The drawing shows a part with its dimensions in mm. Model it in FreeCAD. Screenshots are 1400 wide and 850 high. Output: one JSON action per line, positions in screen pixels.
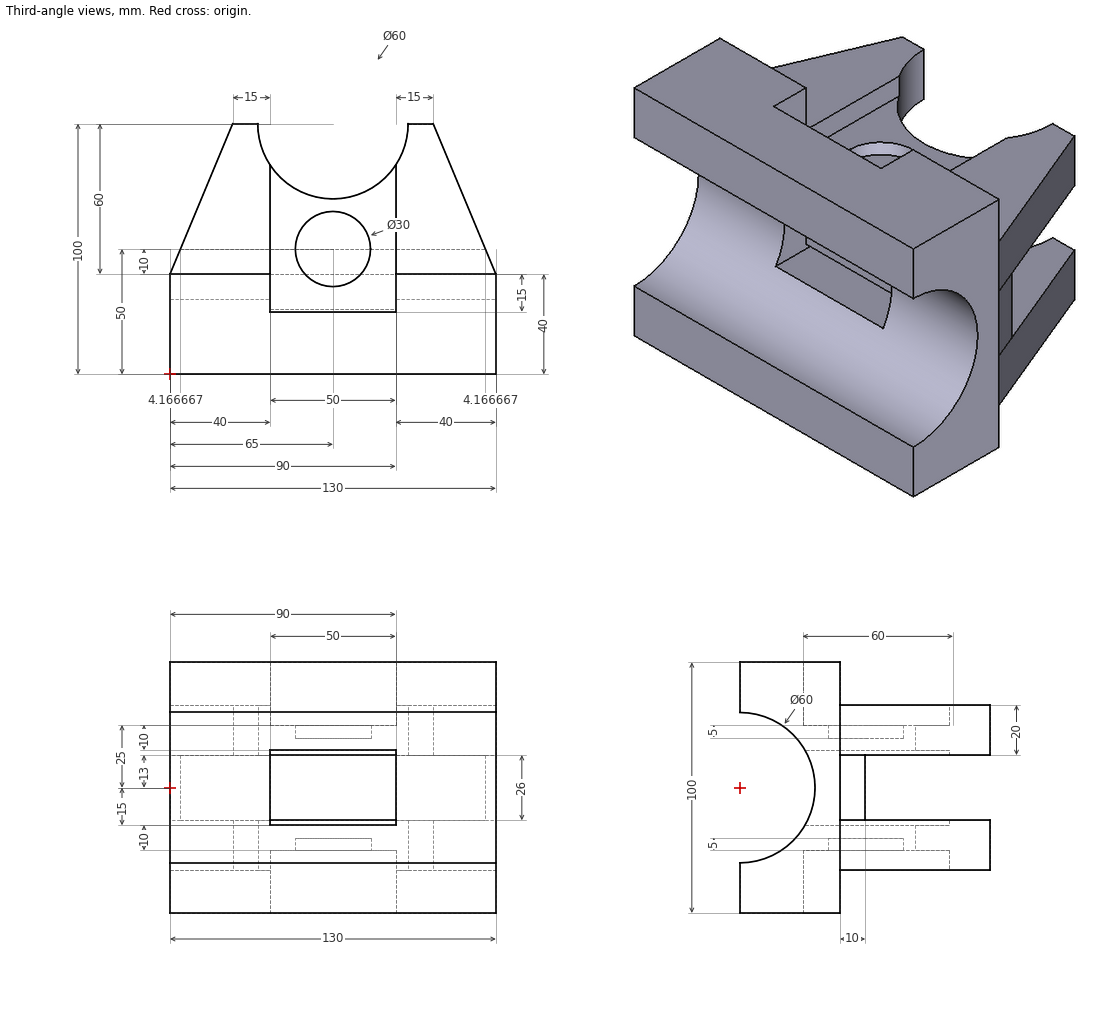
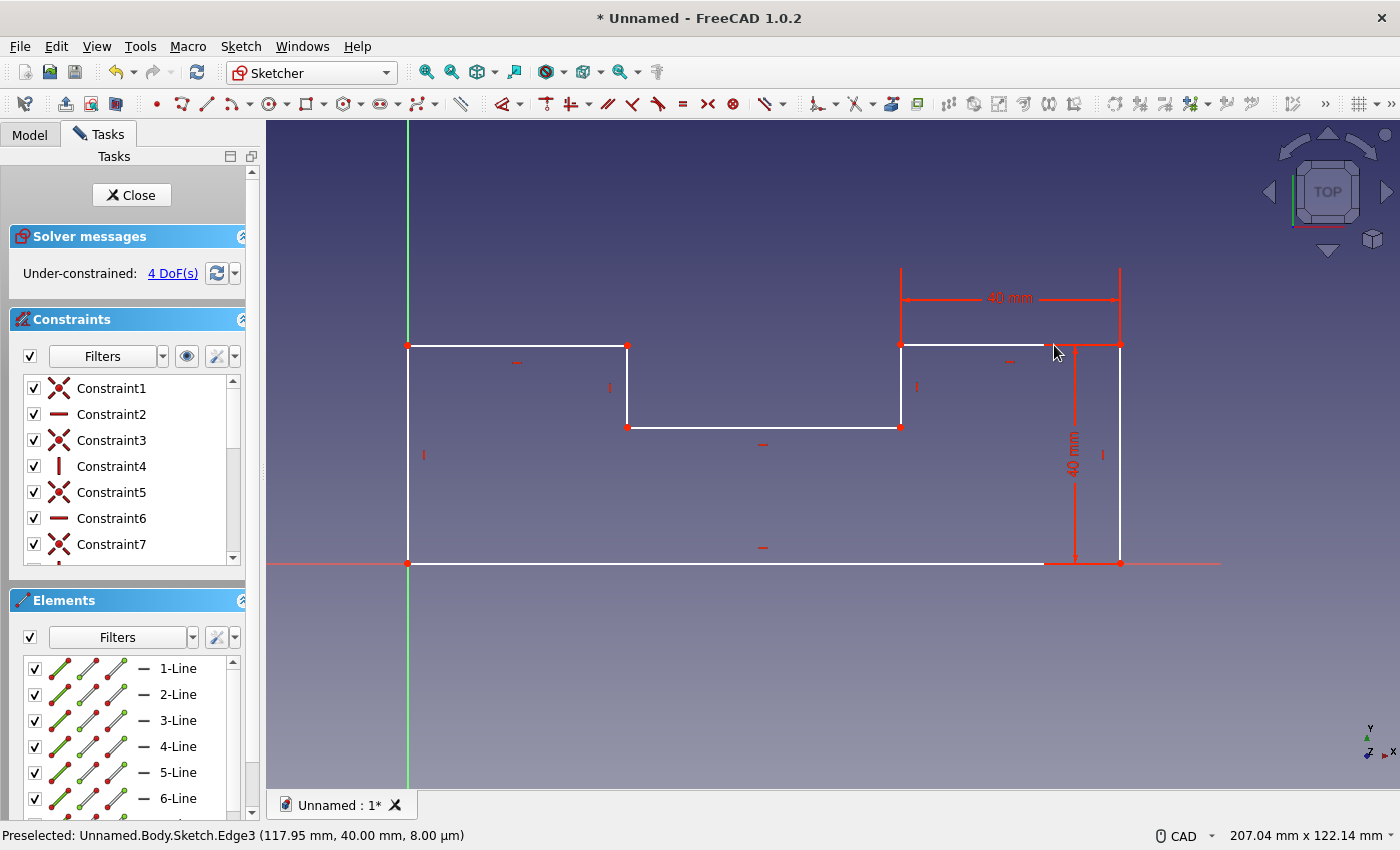
{"action": "left_click", "coordinate": [901, 370]}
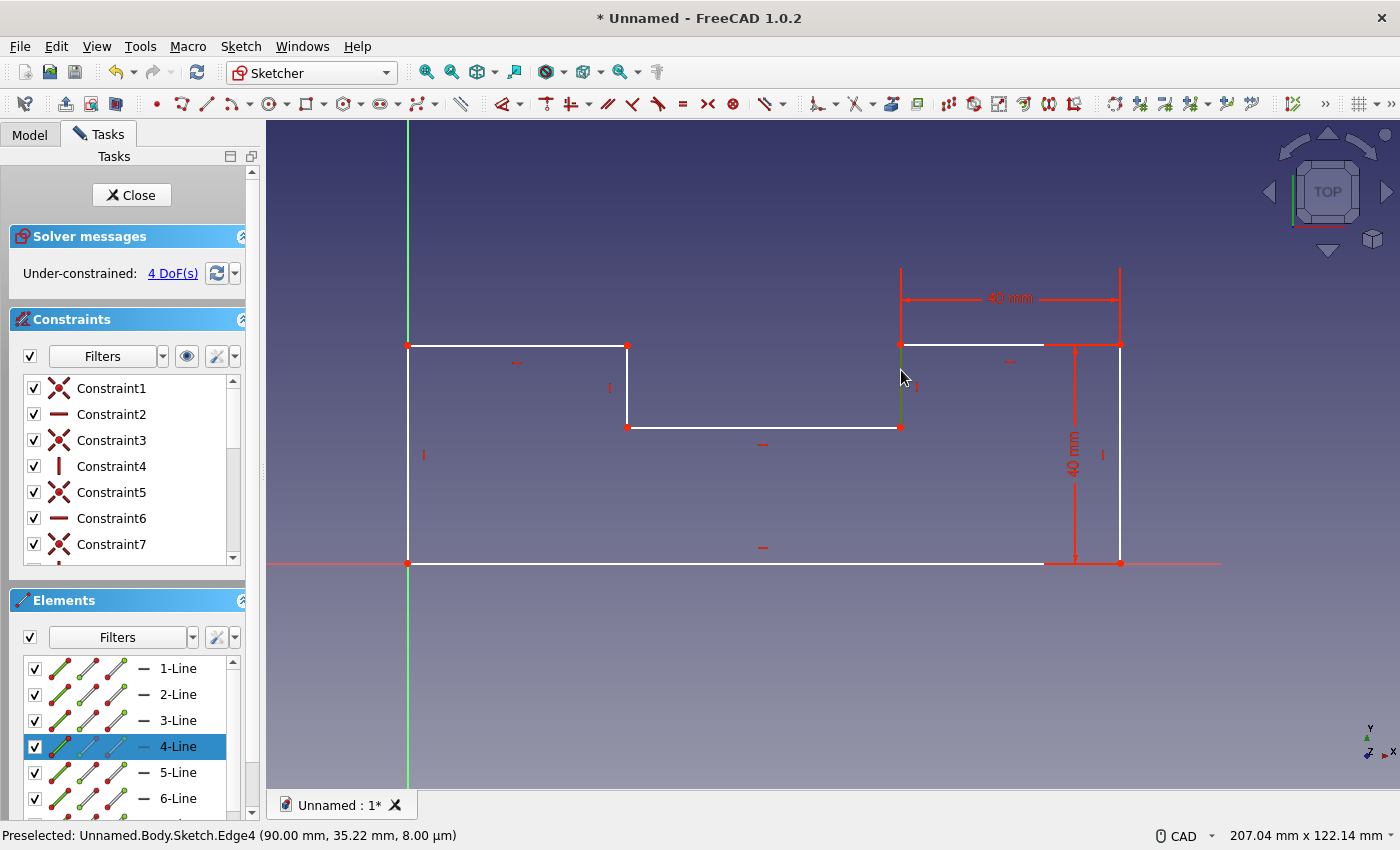
{"action": "left_click", "coordinate": [520, 104]}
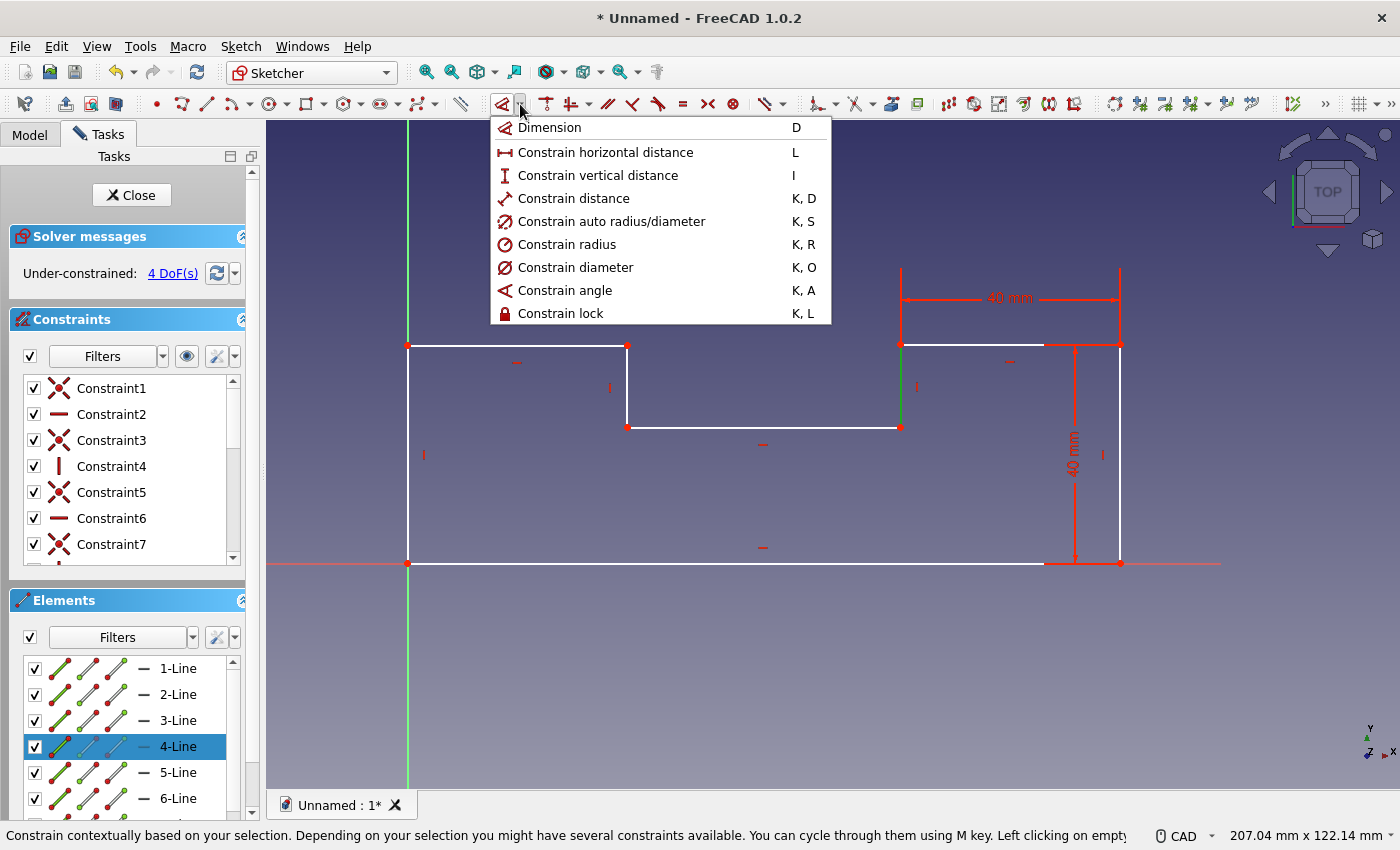
{"action": "left_click", "coordinate": [661, 176]}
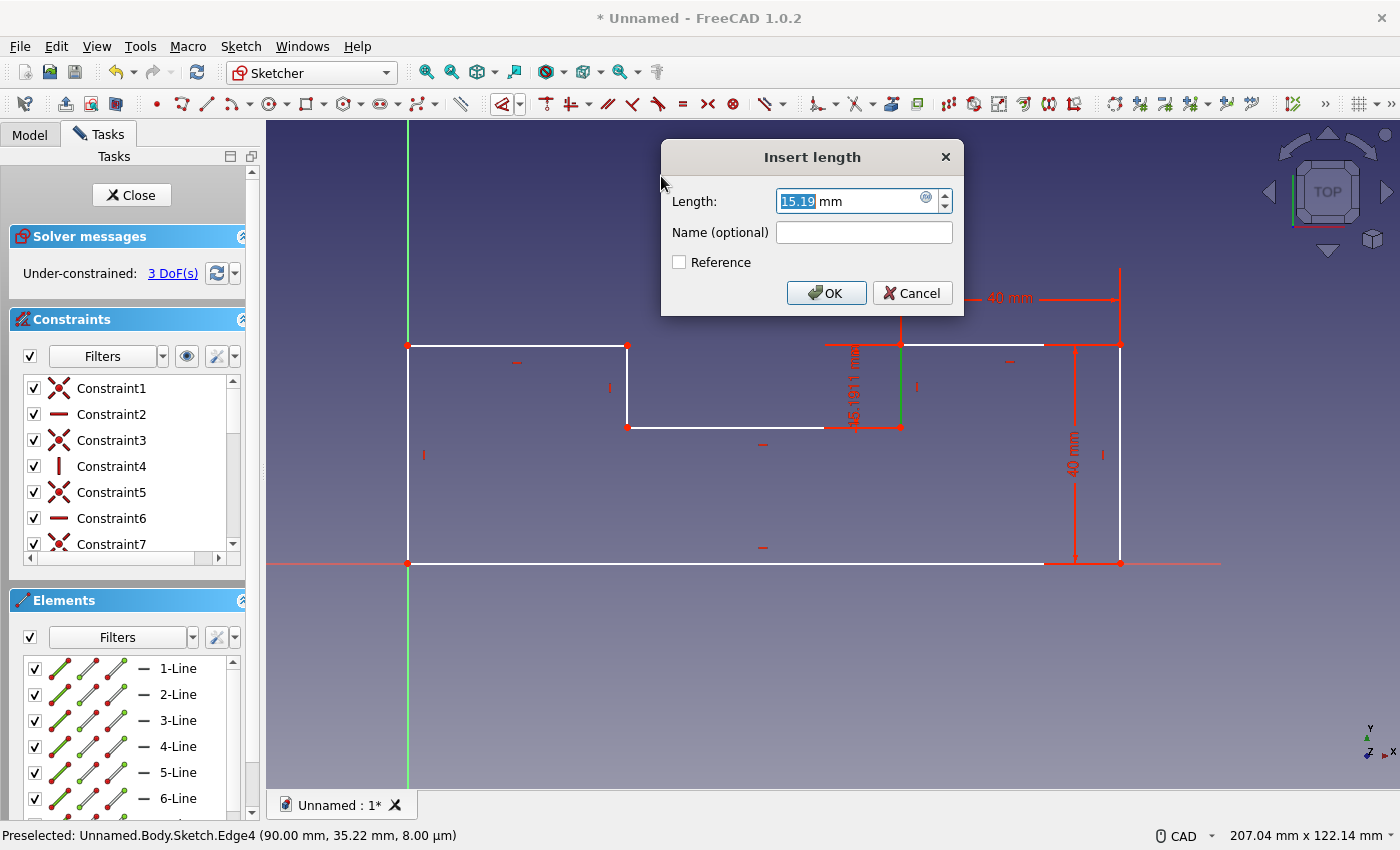
{"action": "type", "text": "15"}
{"action": "key", "text": "Return"}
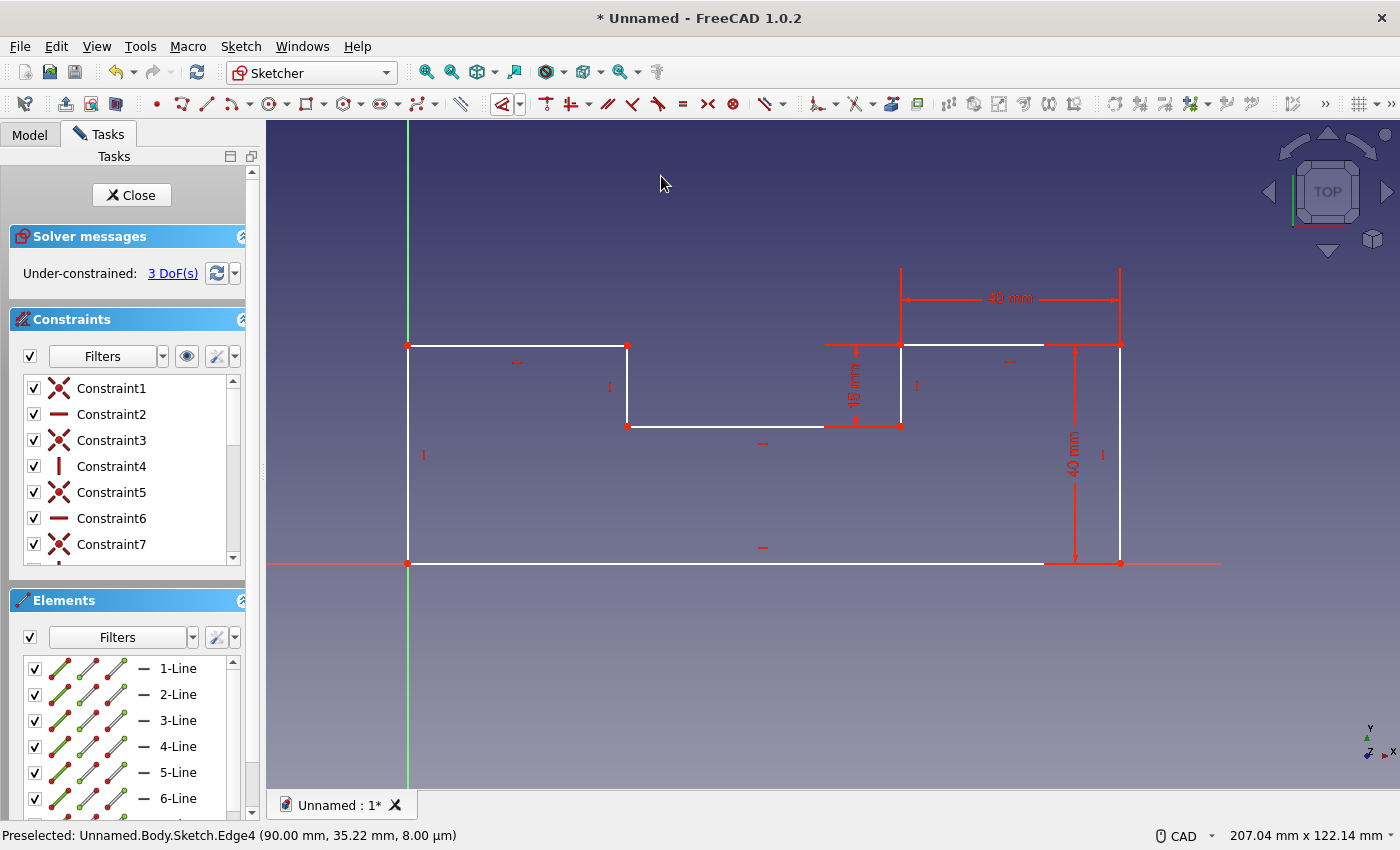
{"action": "left_click", "coordinate": [819, 427]}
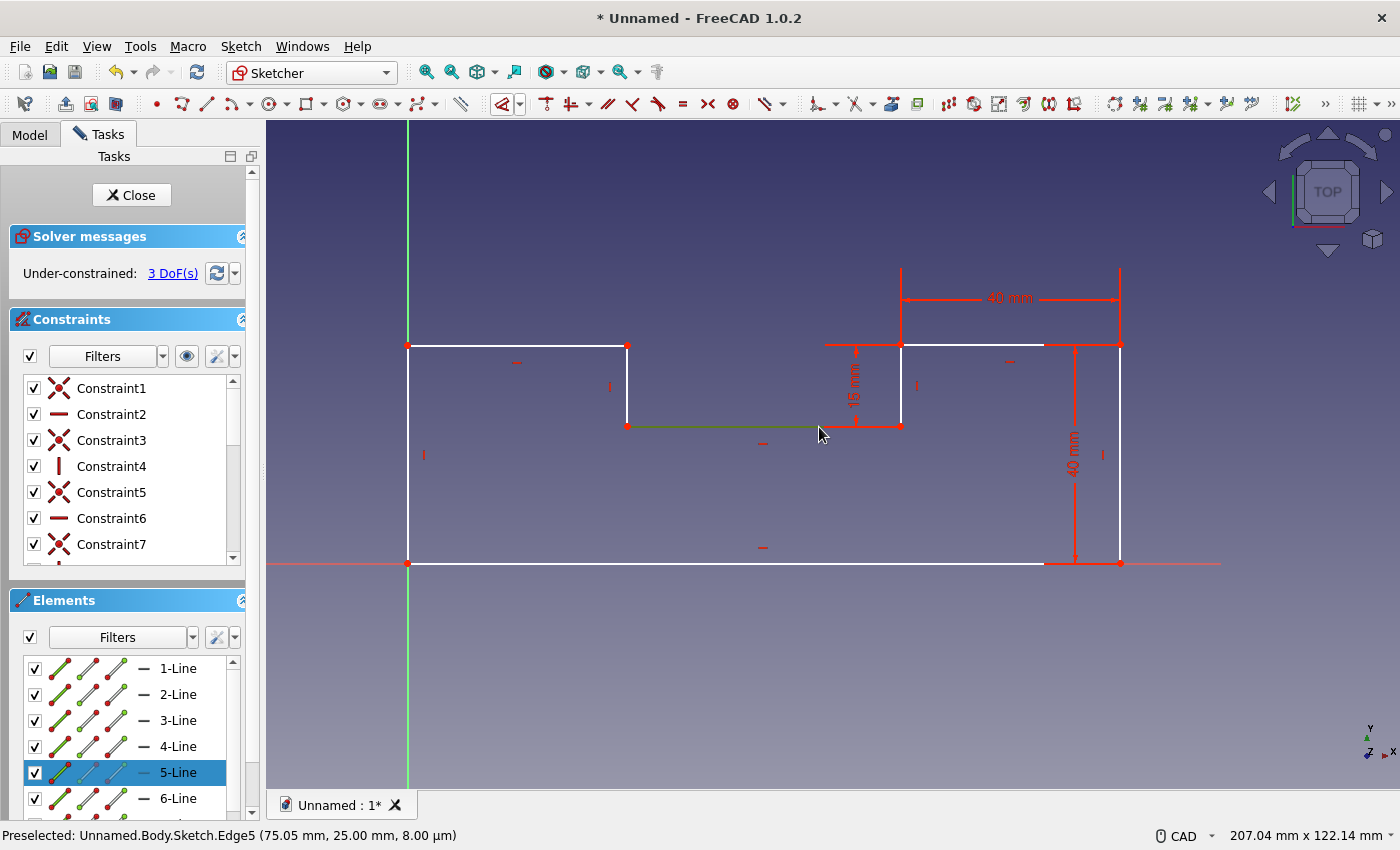
{"action": "left_click", "coordinate": [520, 104]}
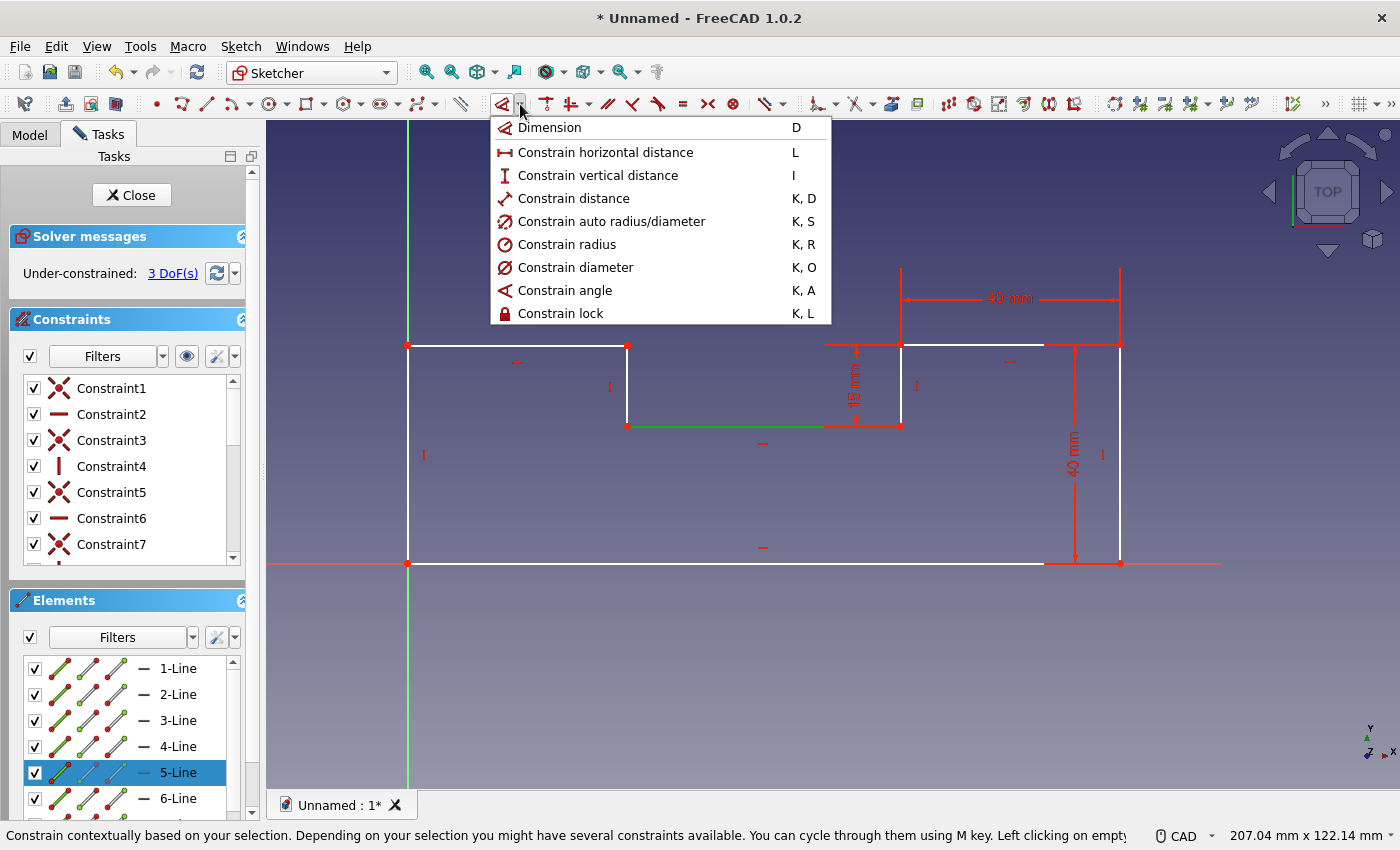
{"action": "left_click", "coordinate": [661, 152]}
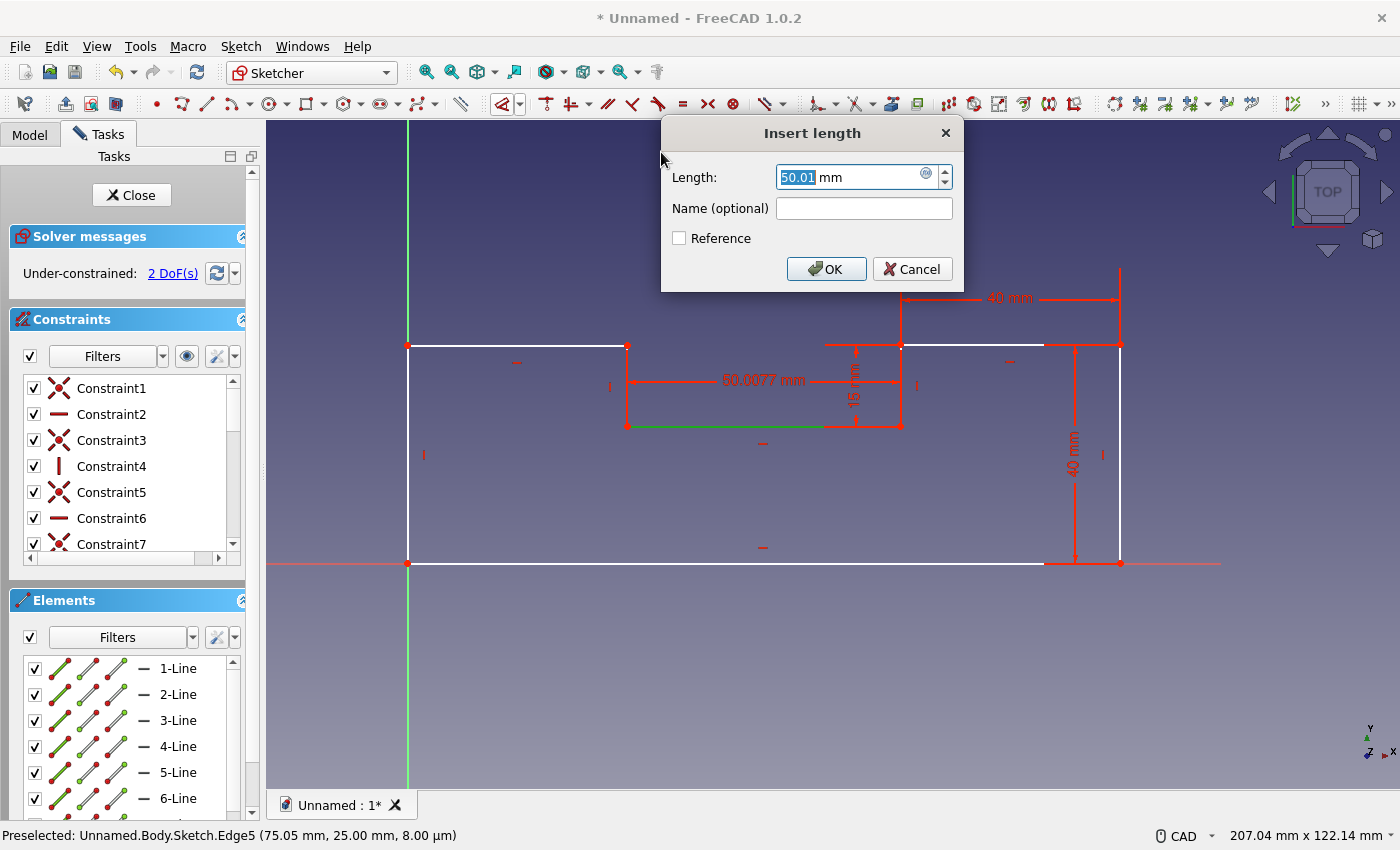
{"action": "type", "text": "50"}
{"action": "key", "text": "Return"}